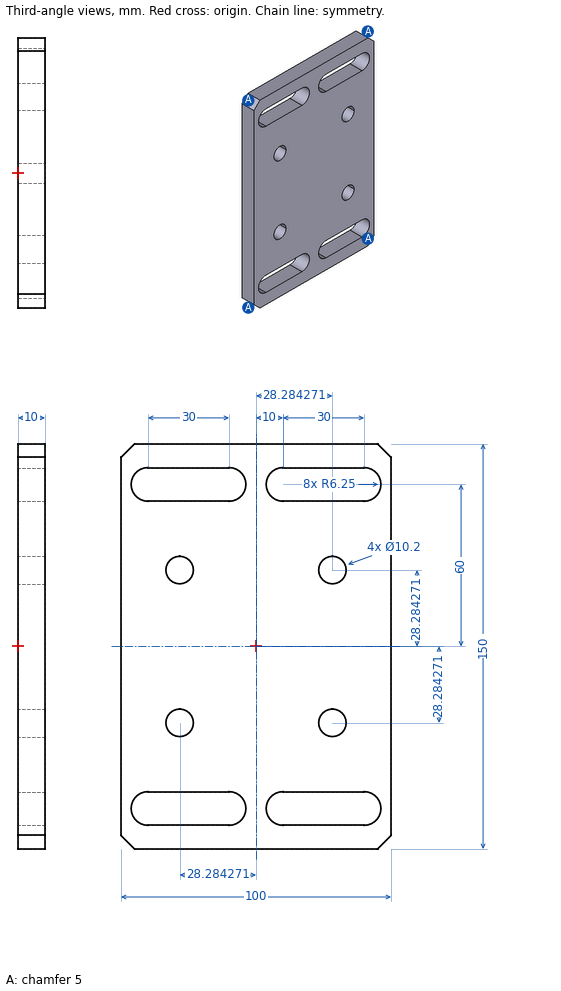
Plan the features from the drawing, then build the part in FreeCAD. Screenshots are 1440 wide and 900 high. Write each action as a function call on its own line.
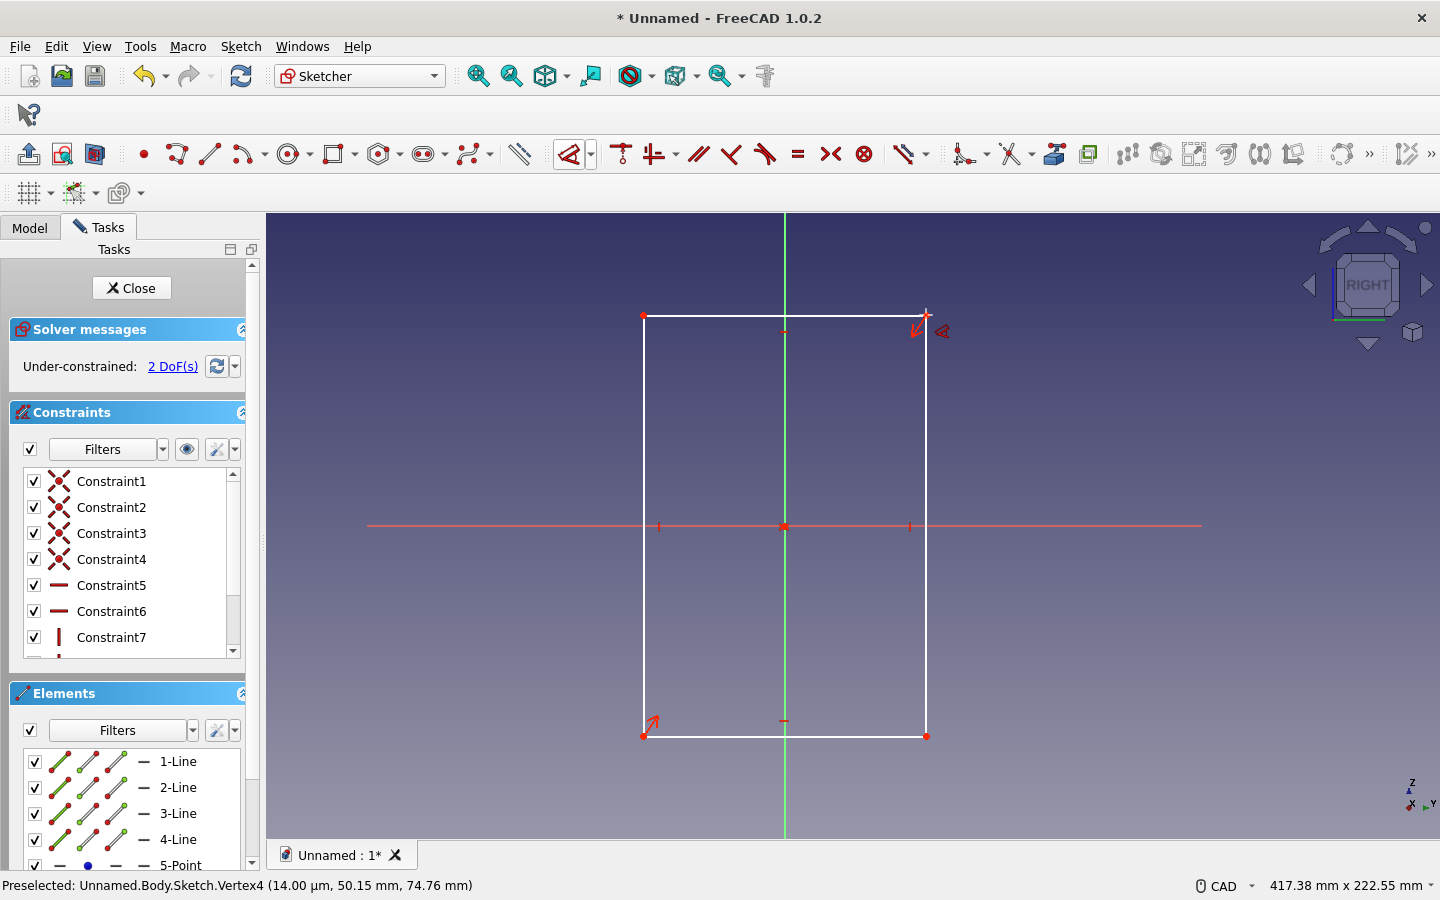
click(729, 737)
click(720, 771)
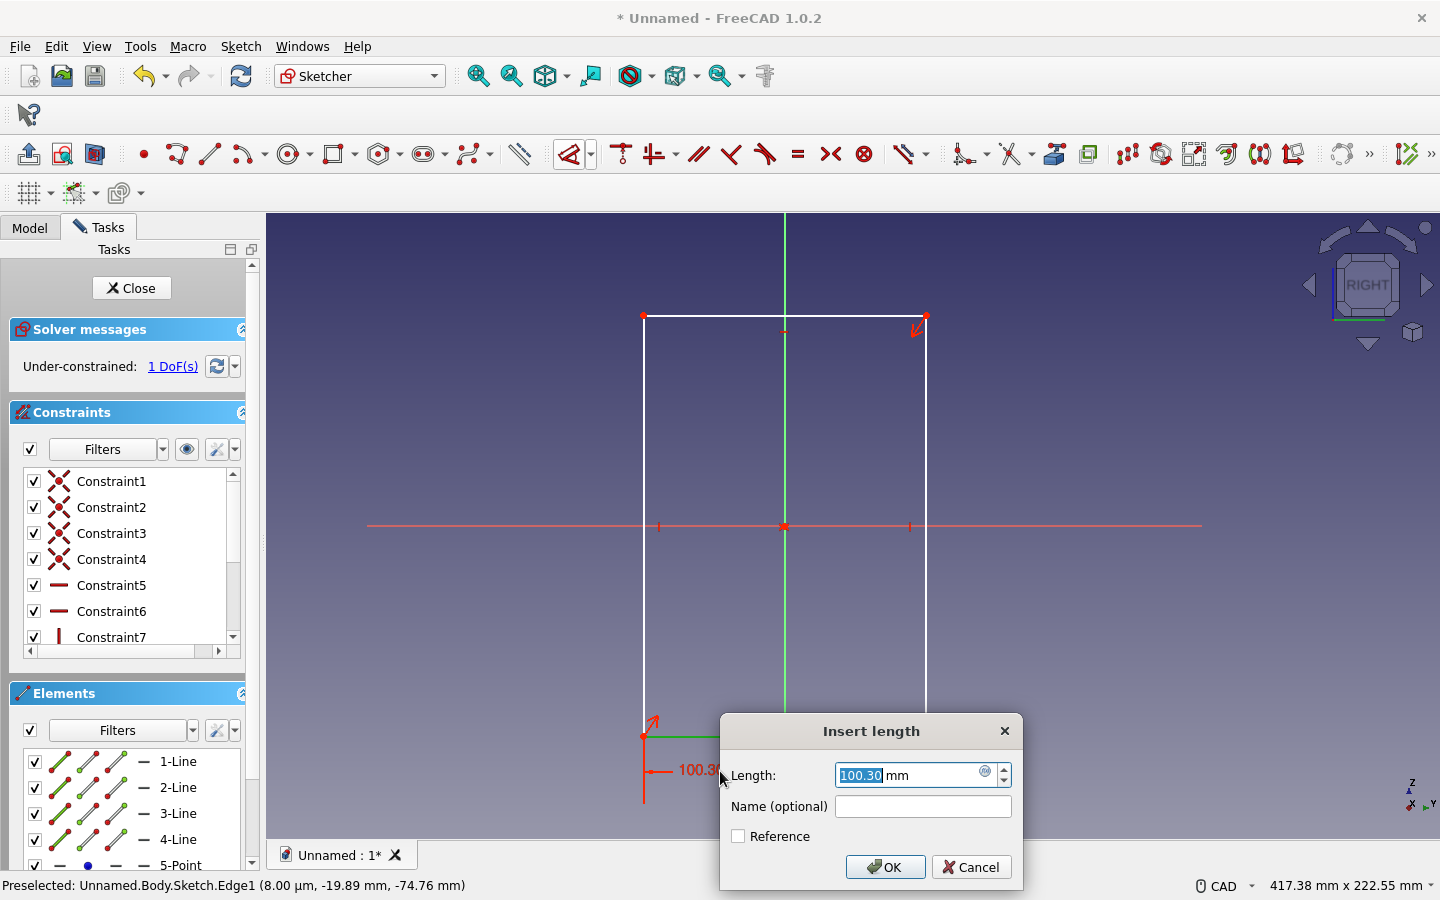
text(100)
key(Return)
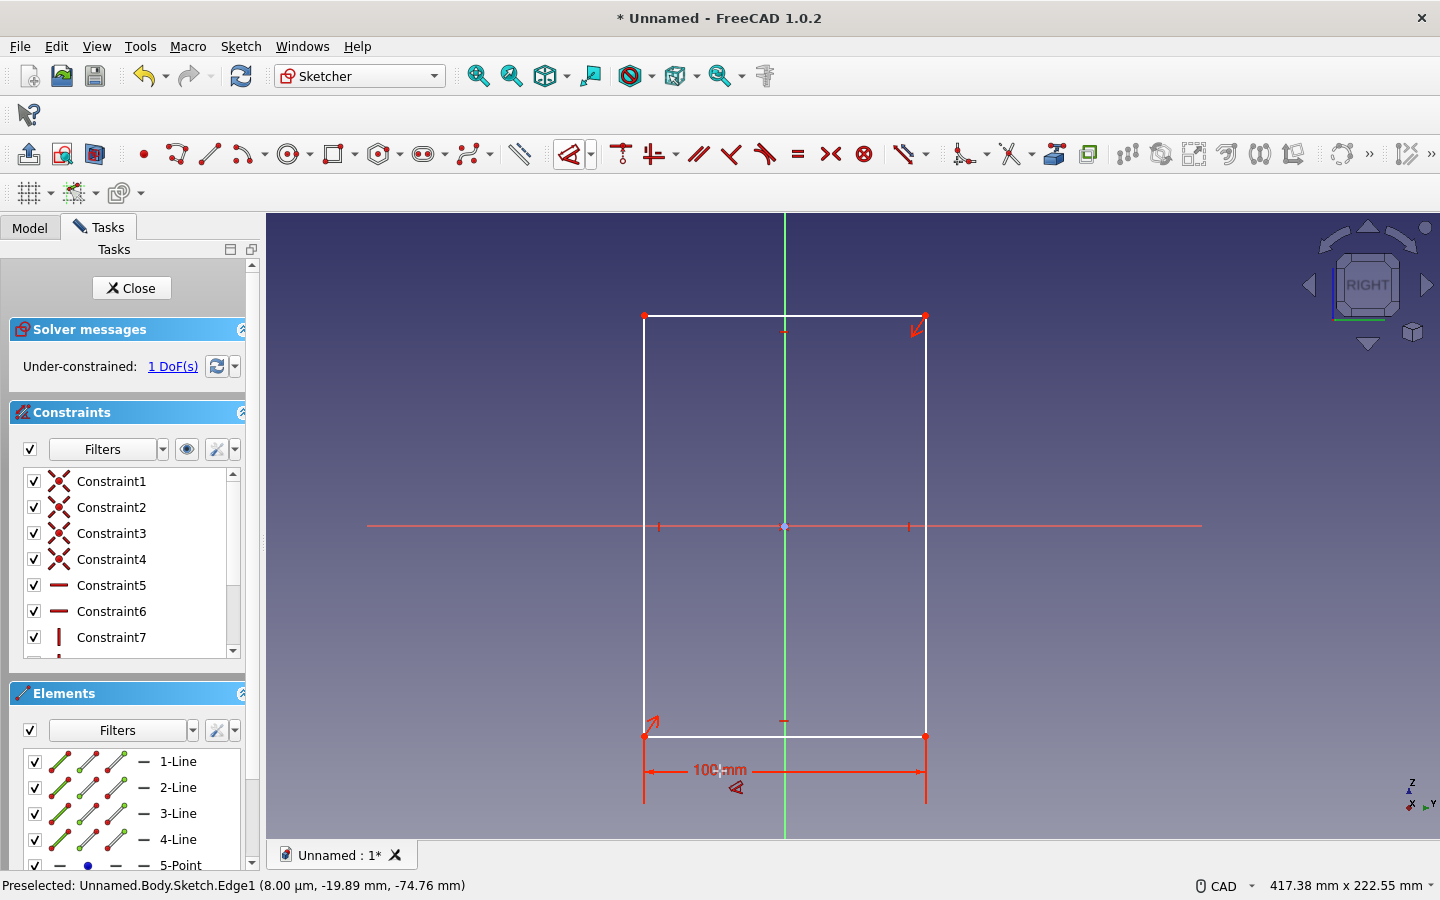
click(926, 610)
click(960, 430)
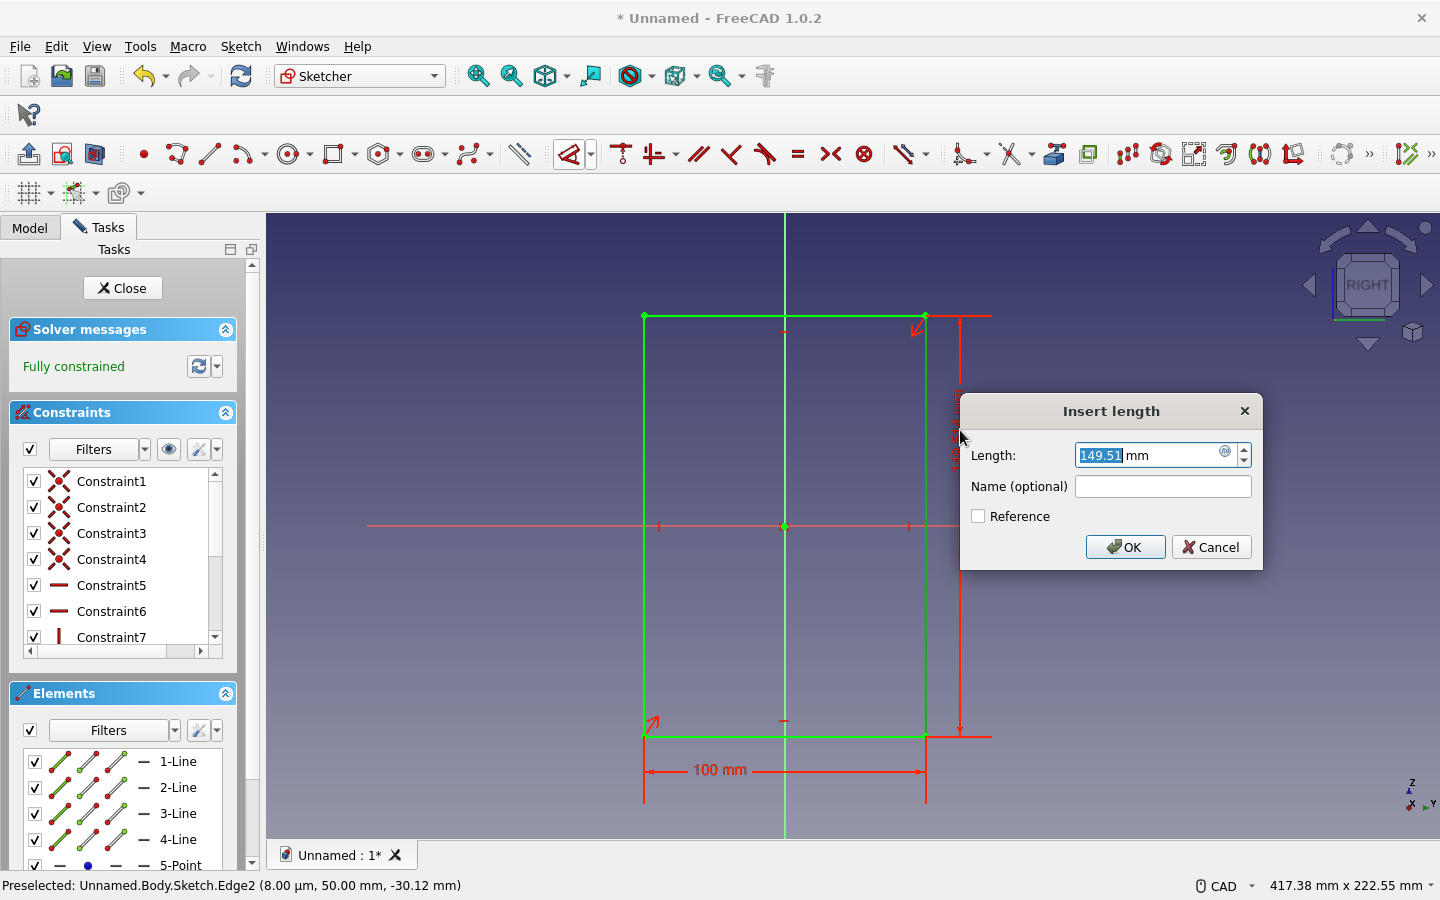
text(150)
key(Return)
key(Escape)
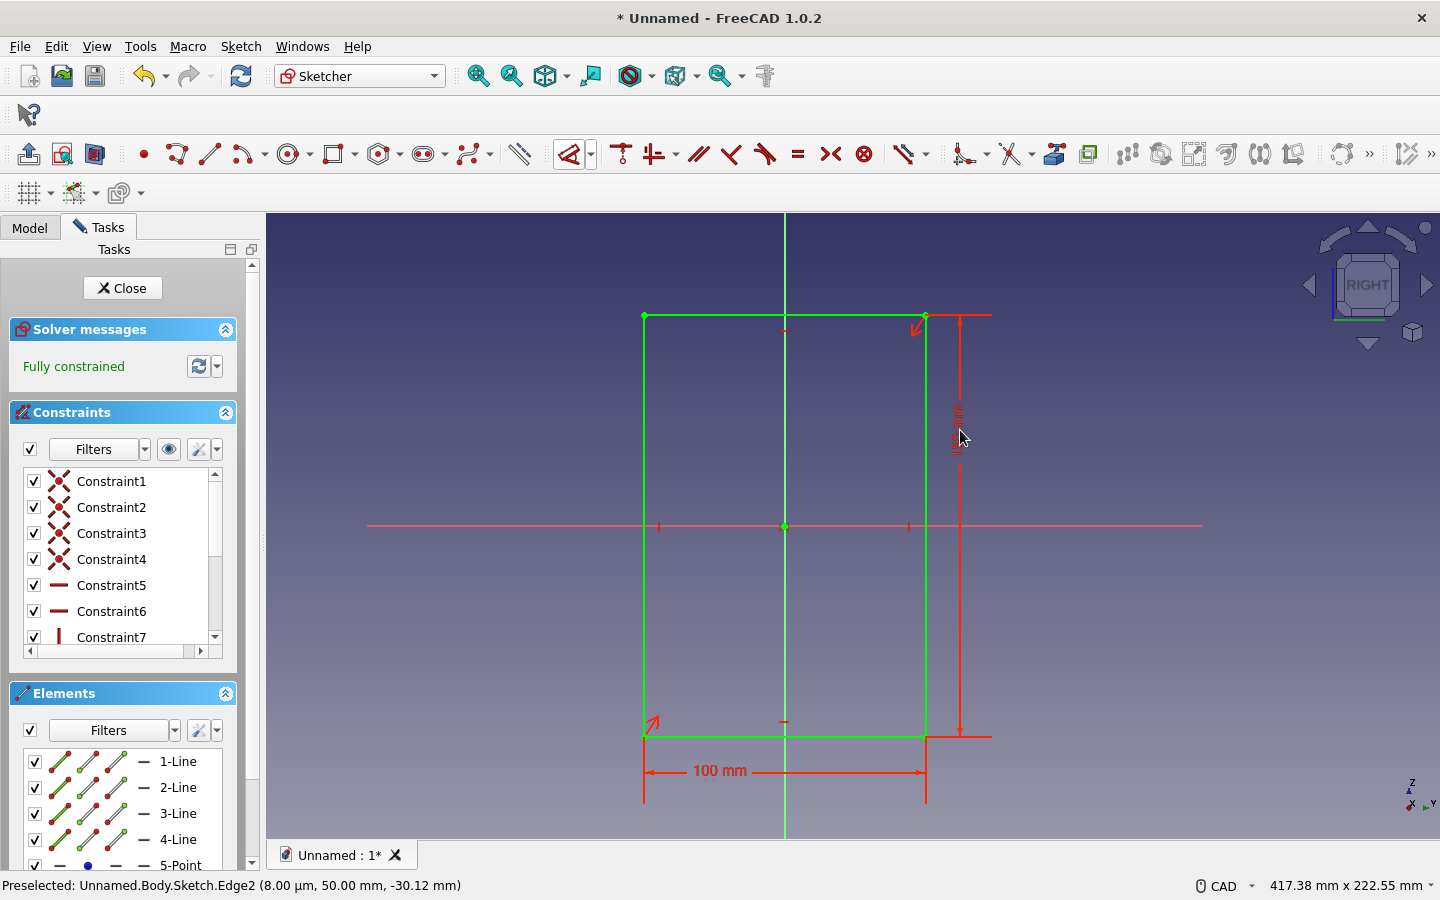
click(123, 288)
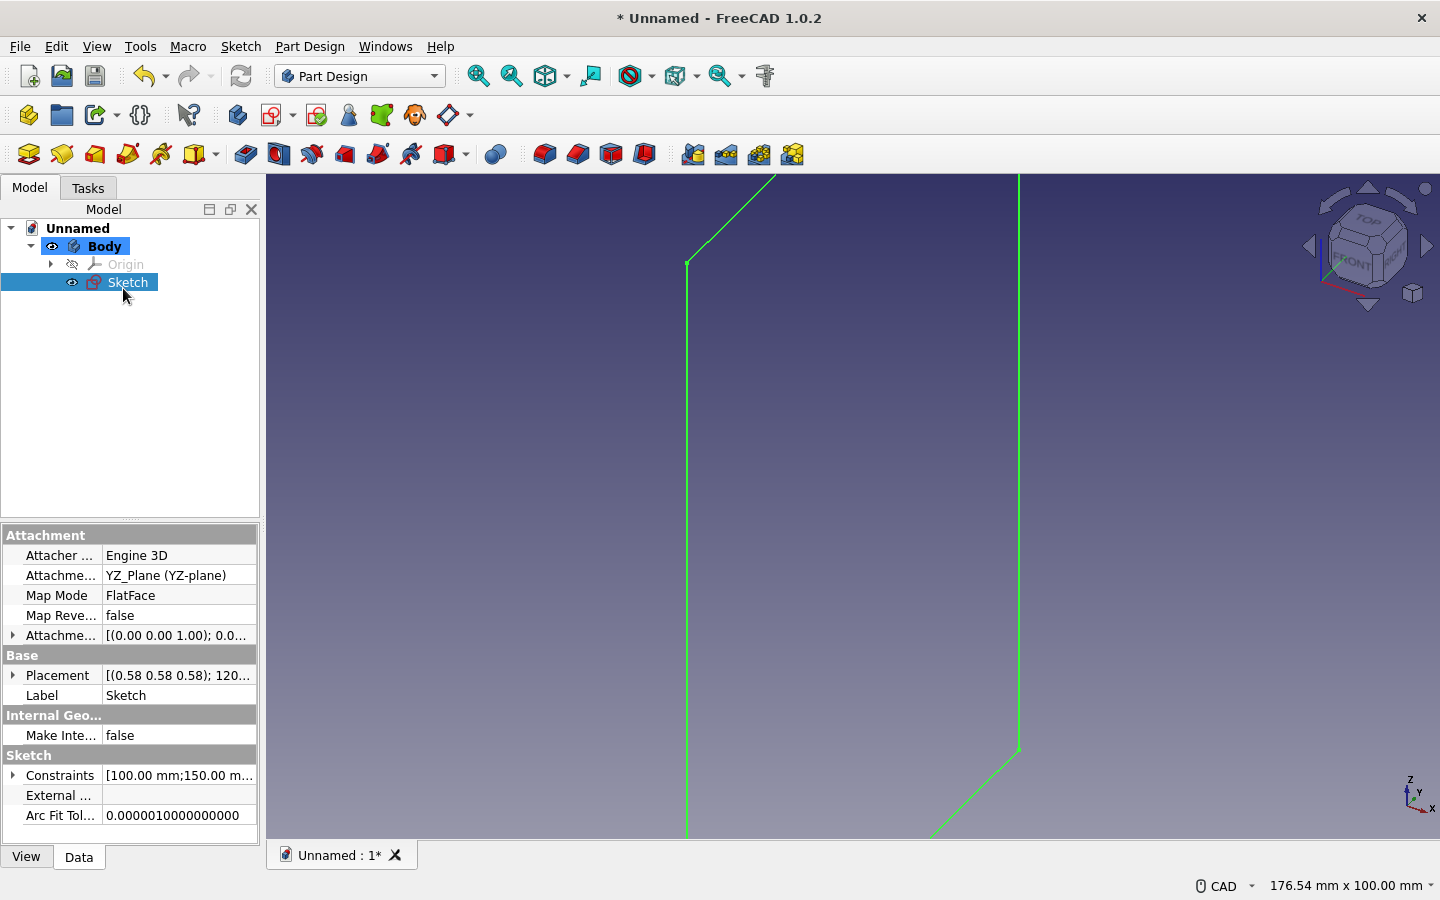
click(29, 154)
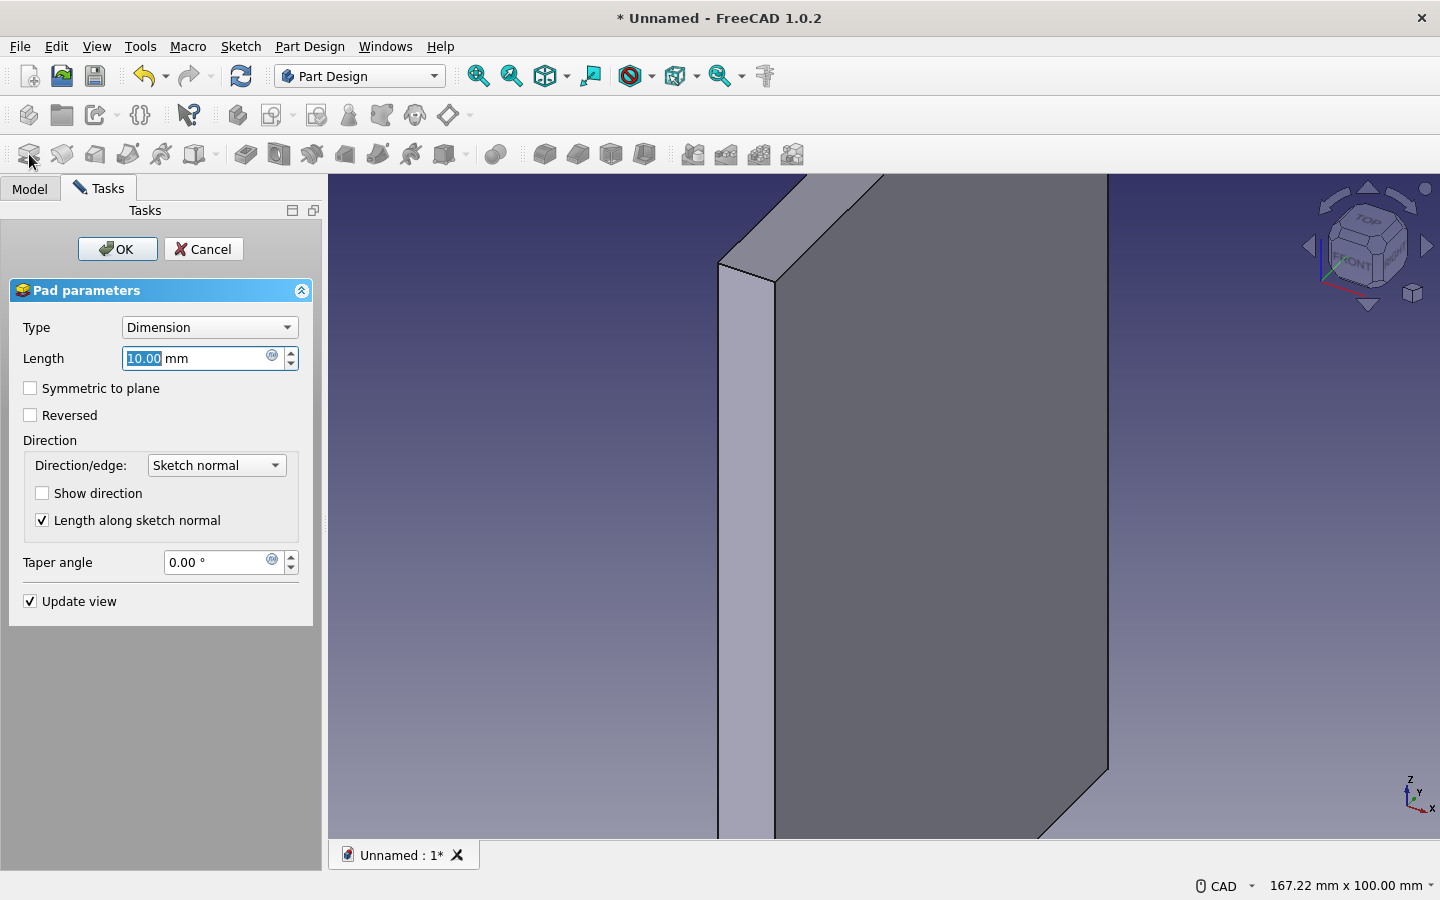
text(10)
key(Tab)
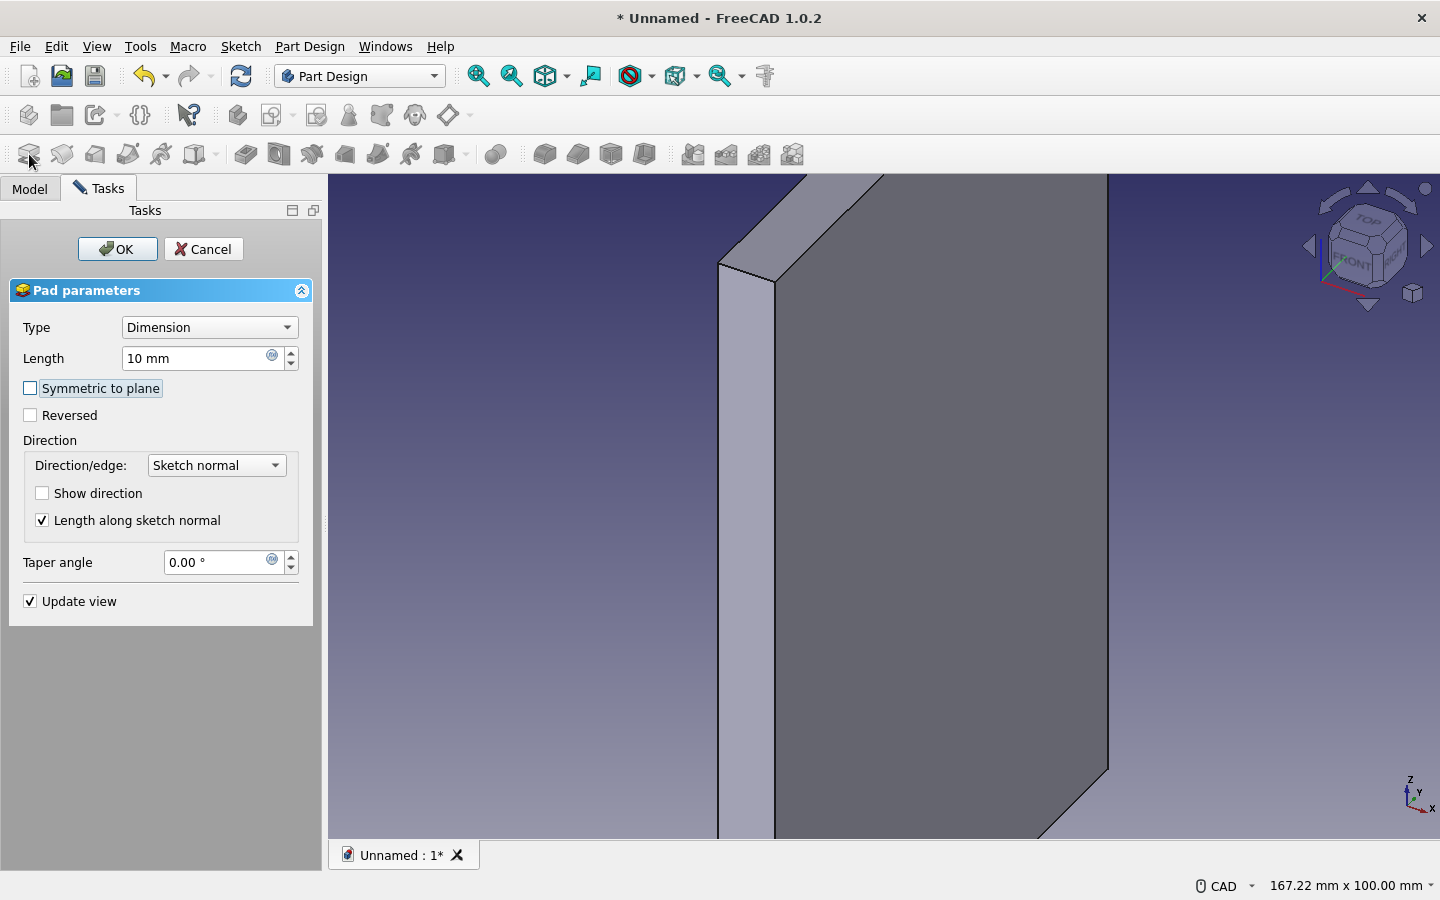
click(118, 249)